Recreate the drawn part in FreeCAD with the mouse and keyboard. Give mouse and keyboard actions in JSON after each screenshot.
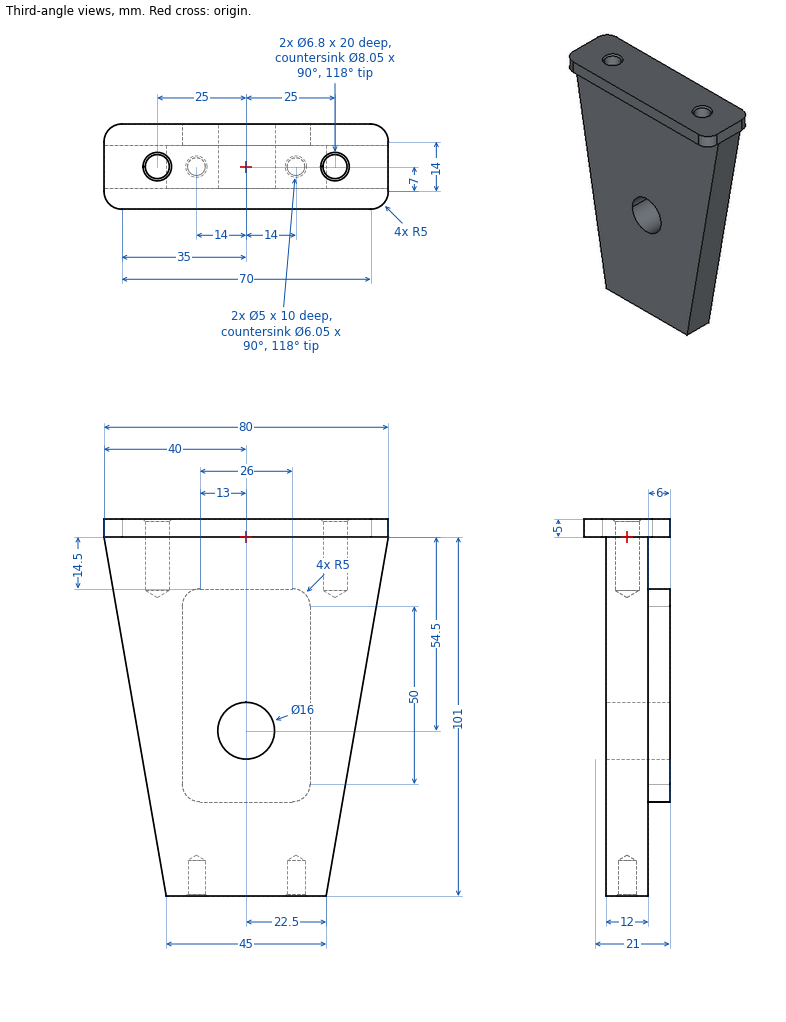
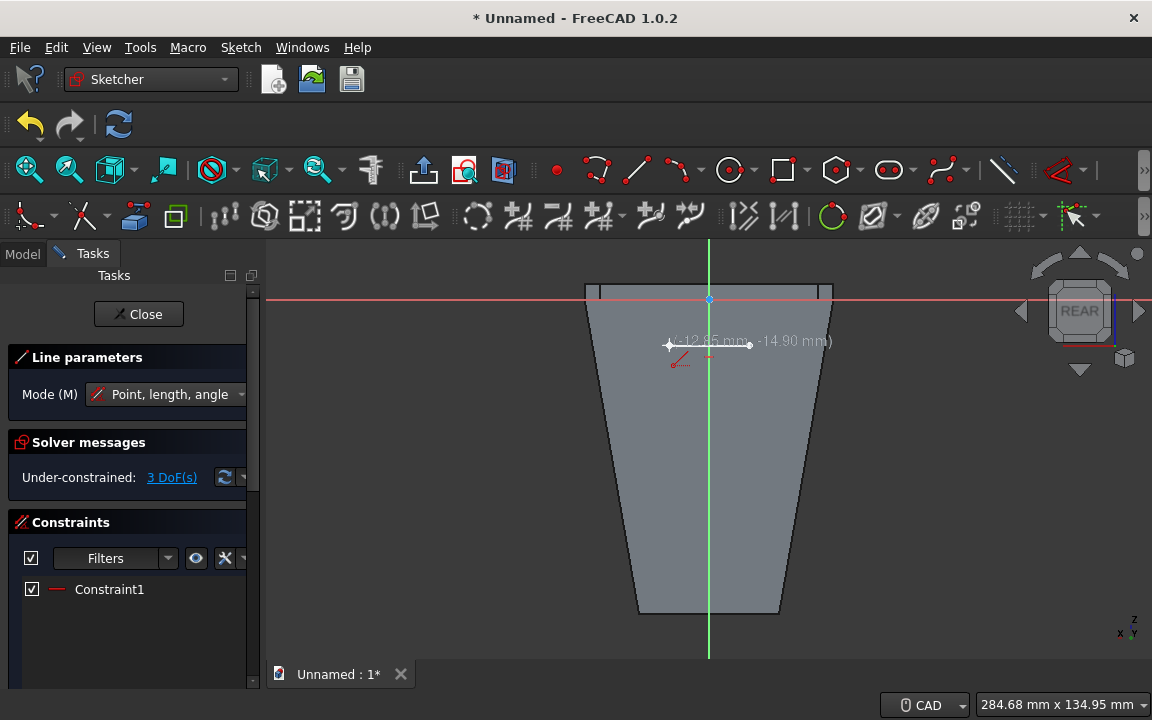
{"action": "left_click", "coordinate": [653, 360]}
{"action": "left_click", "coordinate": [653, 516]}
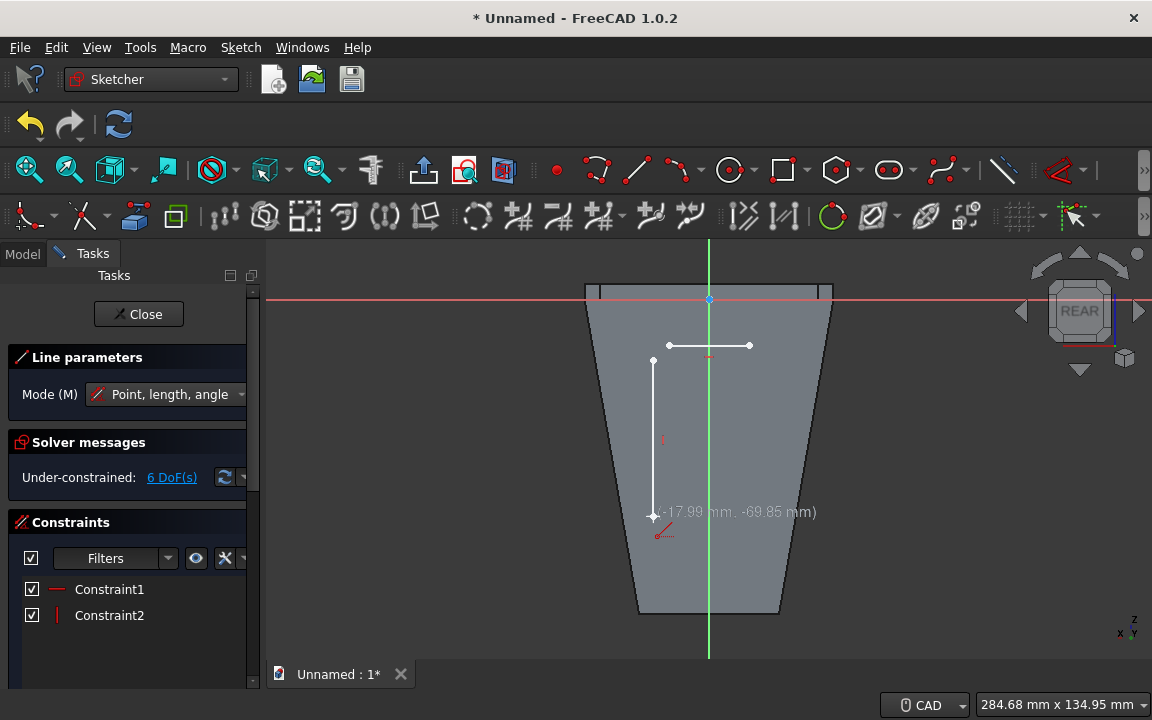
{"action": "left_click", "coordinate": [669, 531]}
{"action": "left_click", "coordinate": [749, 531]}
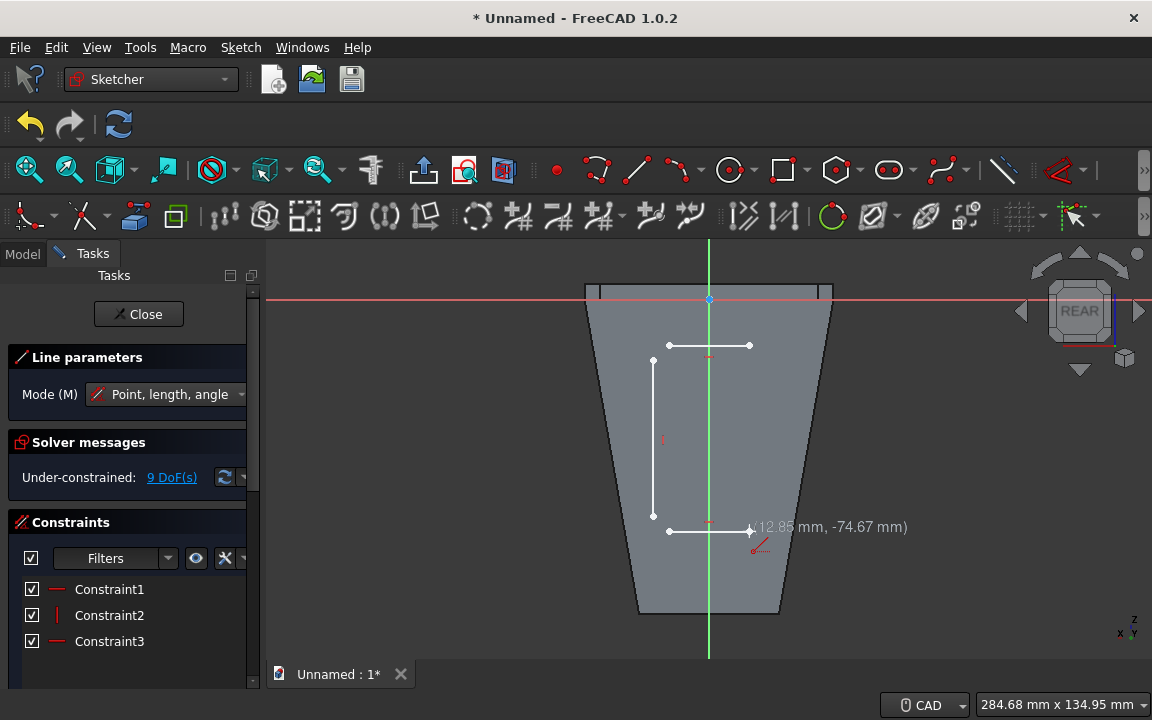
{"action": "left_click", "coordinate": [765, 516]}
{"action": "left_click", "coordinate": [765, 360]}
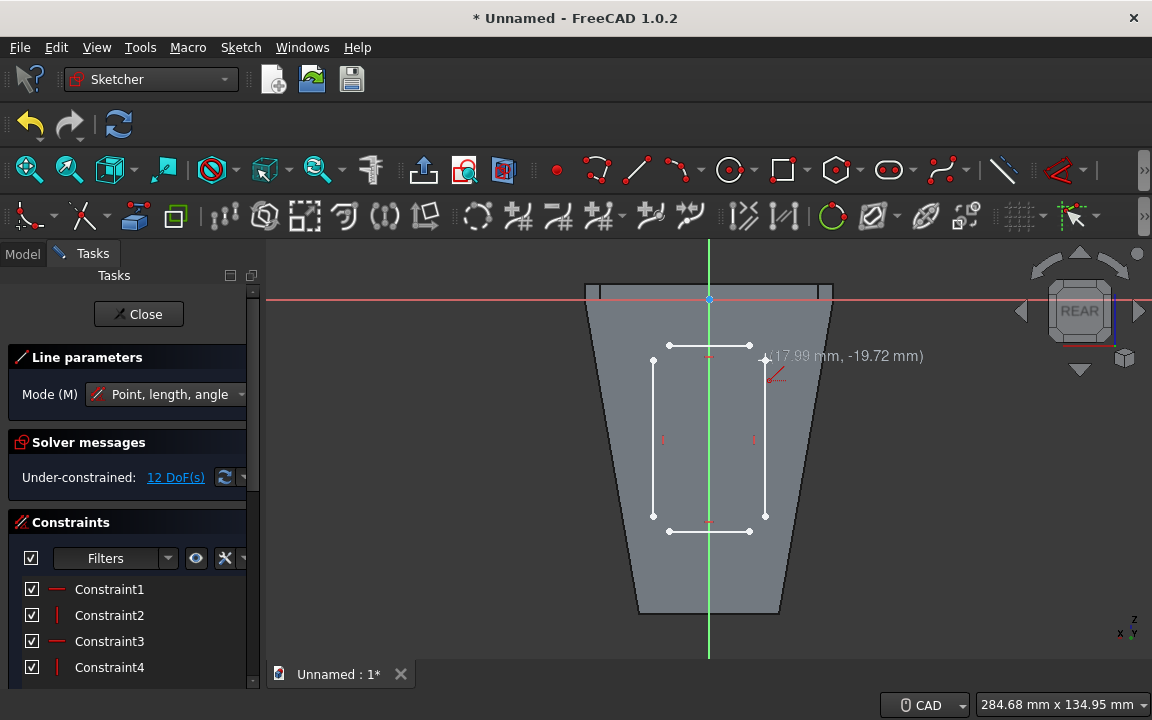
{"action": "key", "text": "g 3 a"}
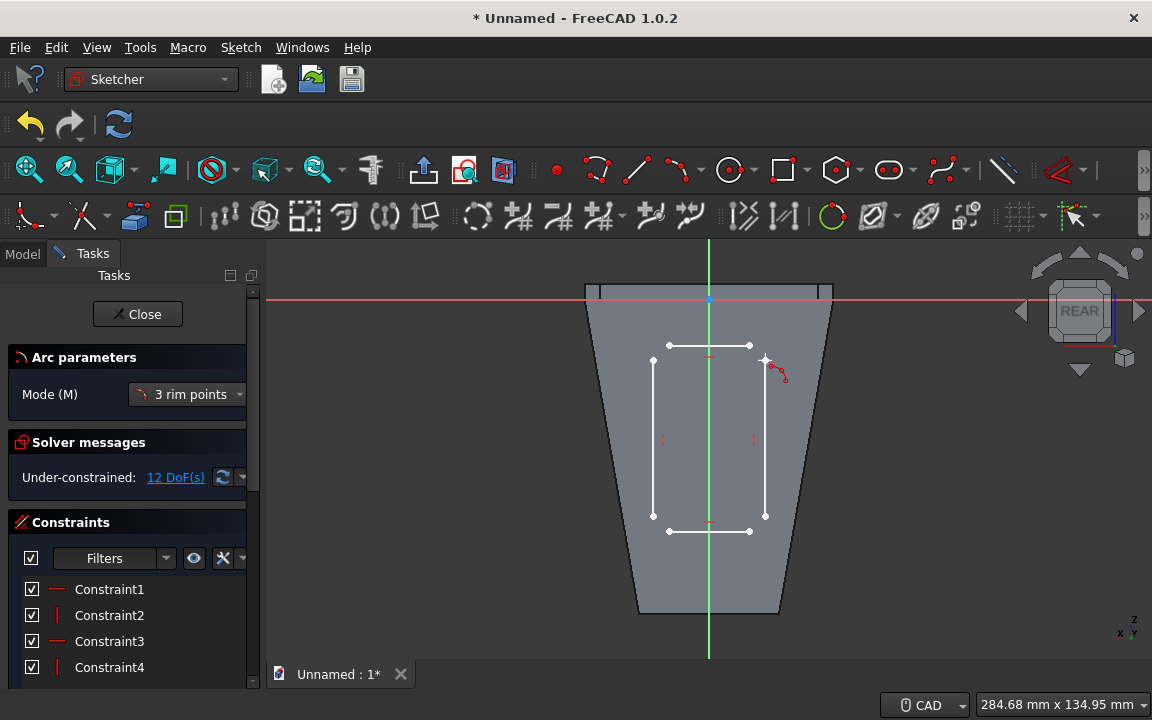
{"action": "left_click", "coordinate": [669, 346]}
{"action": "left_click", "coordinate": [653, 361]}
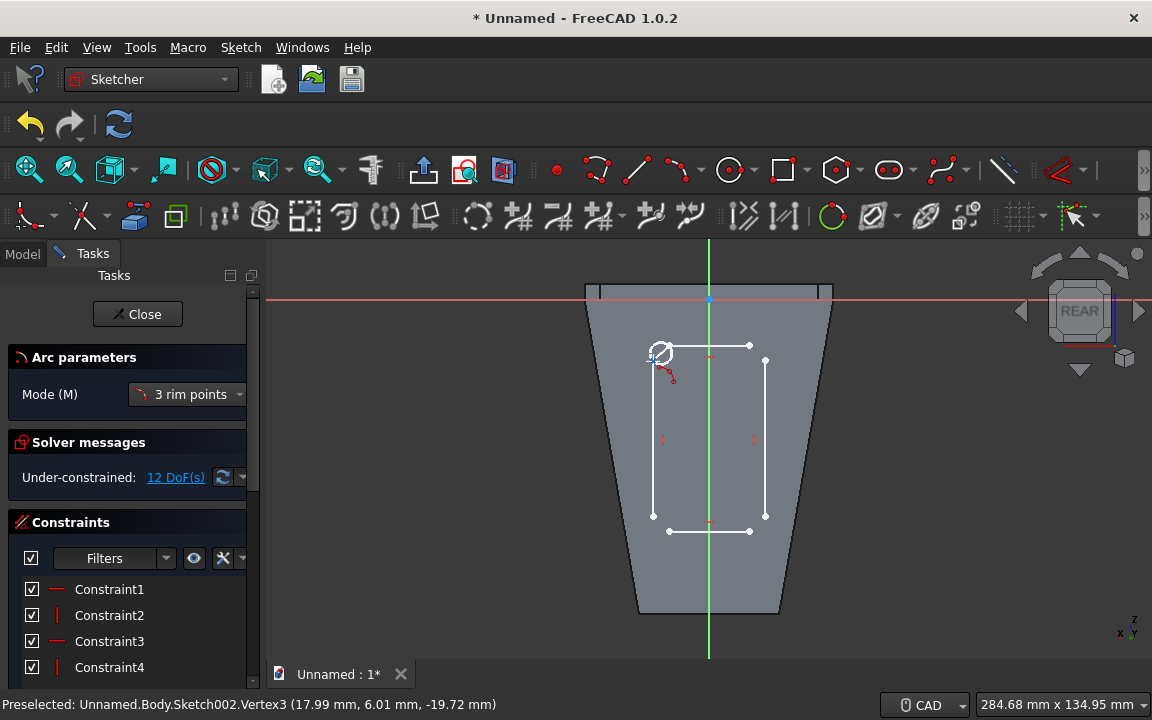
{"action": "scroll", "coordinate": [658, 349], "scroll_direction": "up", "scroll_amount": 7}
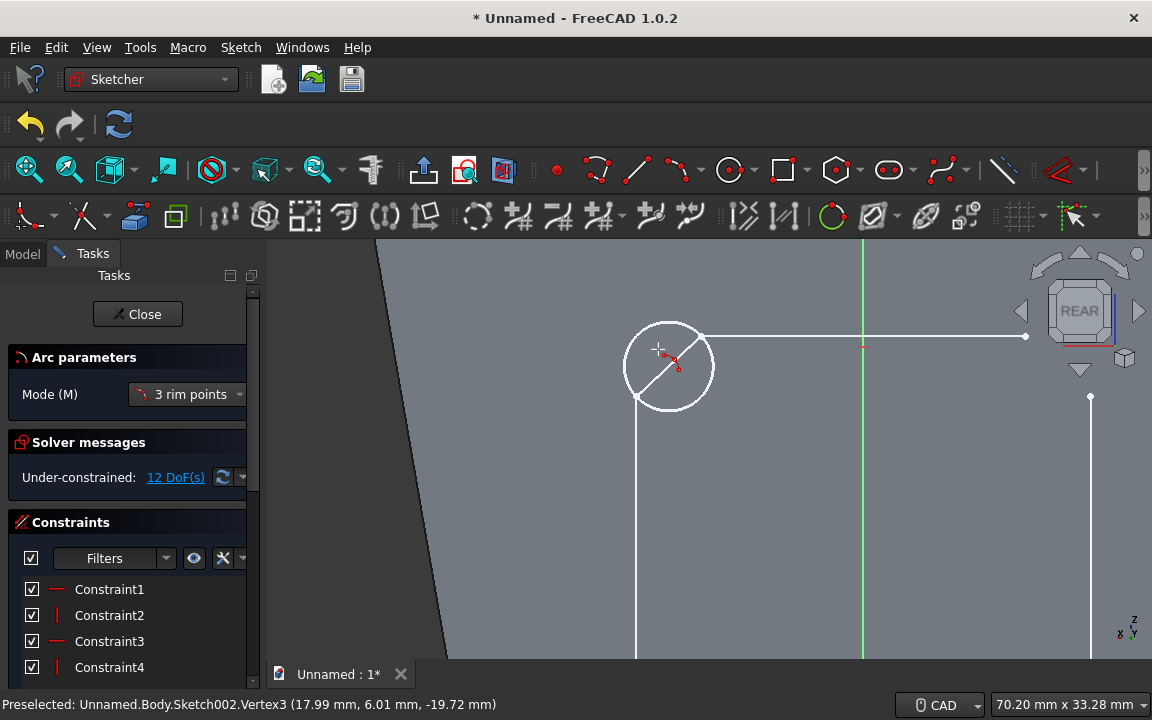
{"action": "left_click", "coordinate": [655, 349]}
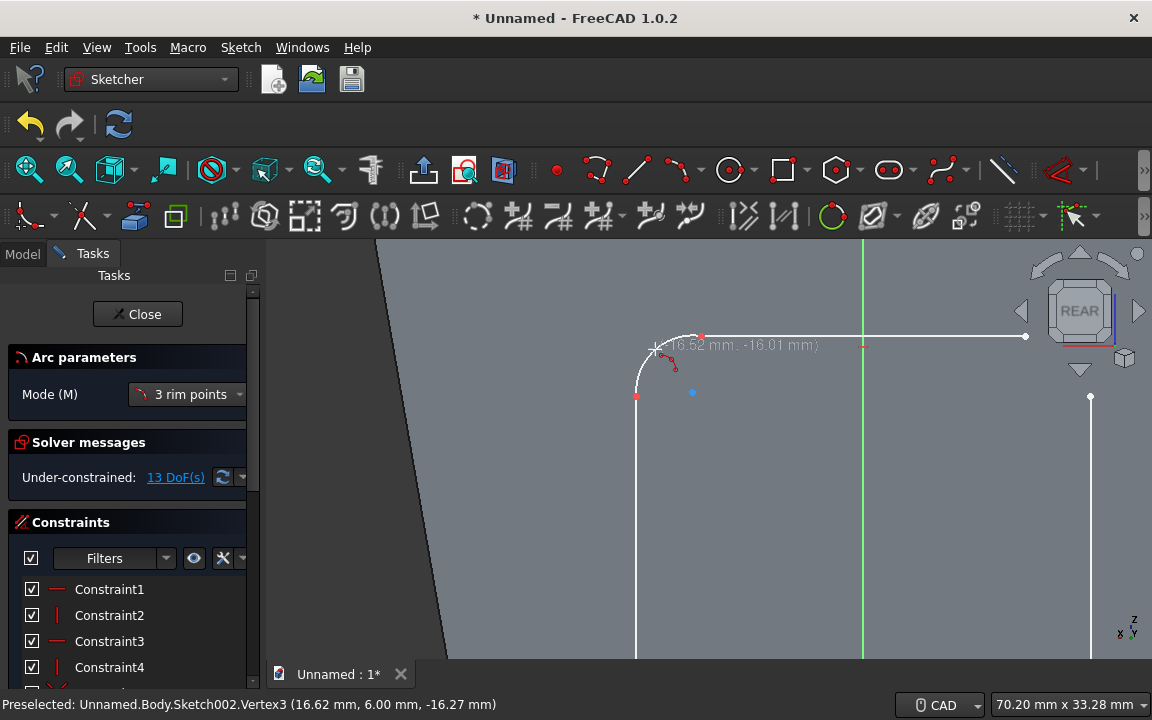
{"action": "scroll", "coordinate": [544, 376], "scroll_direction": "down", "scroll_amount": 6}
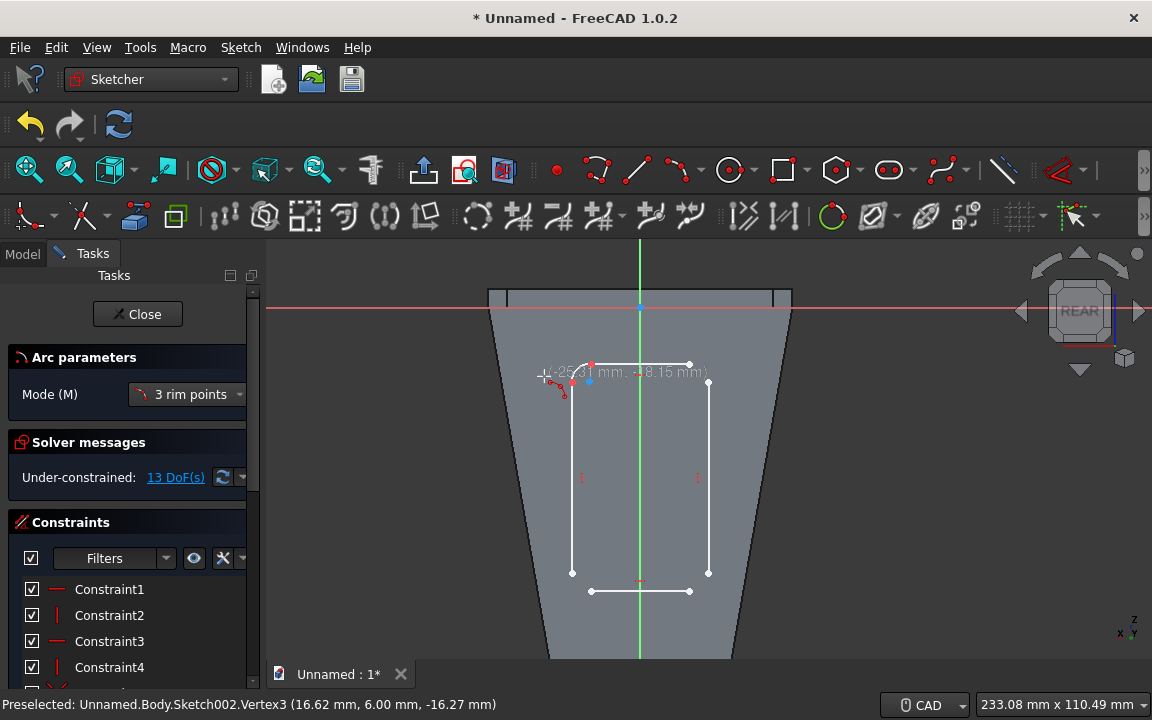
{"action": "left_click", "coordinate": [572, 573]}
{"action": "left_click", "coordinate": [592, 591]}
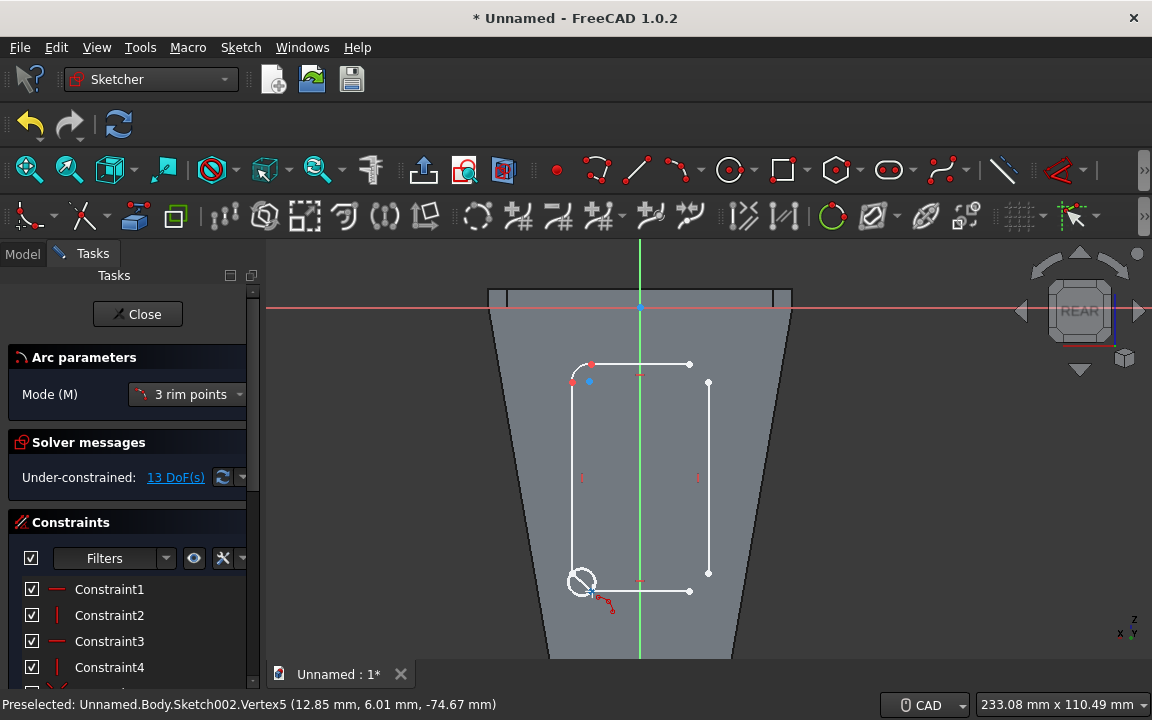
{"action": "scroll", "coordinate": [578, 585], "scroll_direction": "up", "scroll_amount": 6}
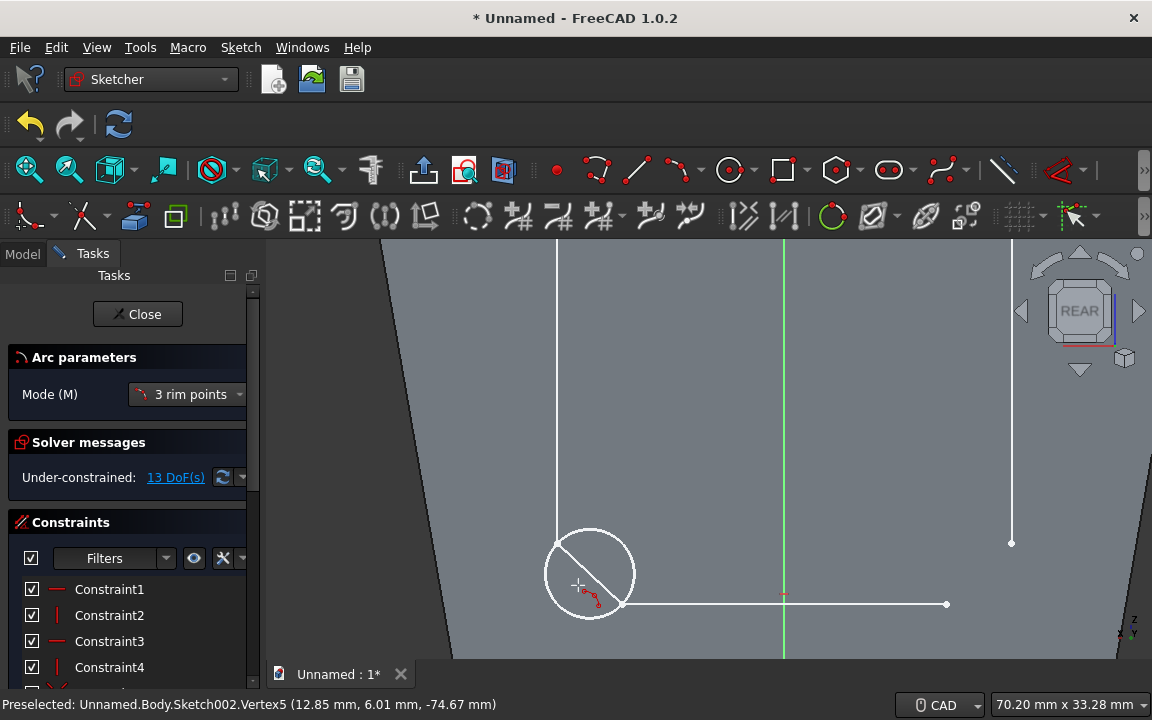
{"action": "left_click", "coordinate": [576, 584]}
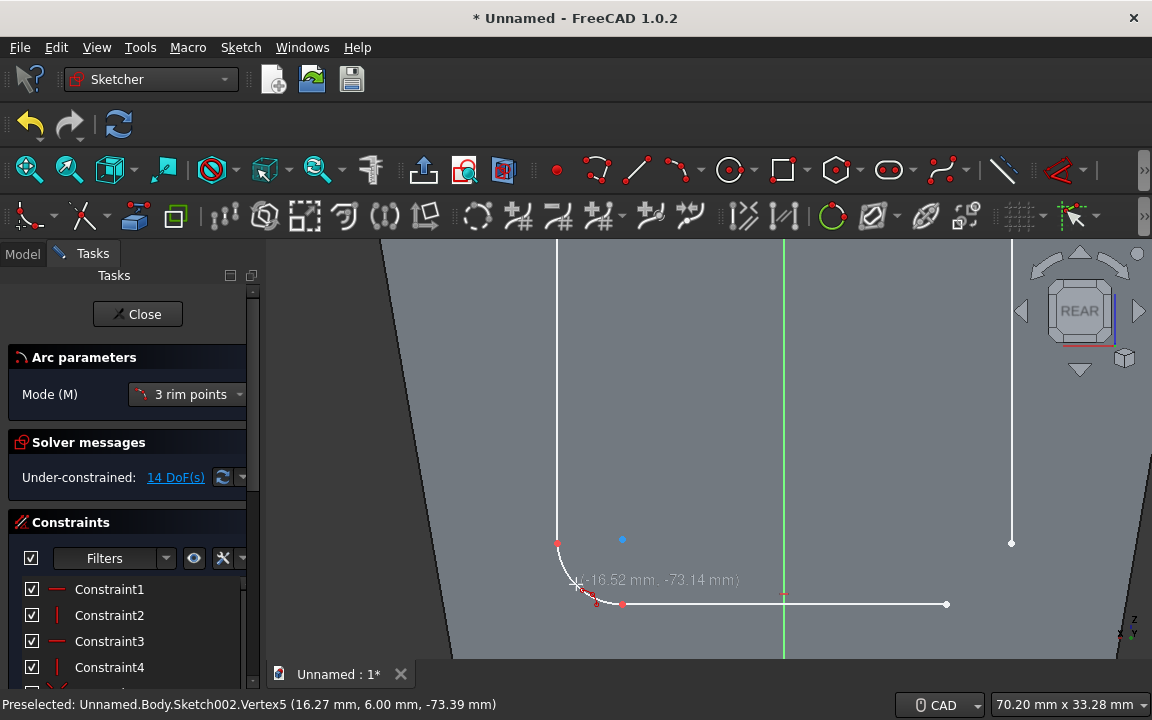
{"action": "scroll", "coordinate": [578, 586], "scroll_direction": "down", "scroll_amount": 6}